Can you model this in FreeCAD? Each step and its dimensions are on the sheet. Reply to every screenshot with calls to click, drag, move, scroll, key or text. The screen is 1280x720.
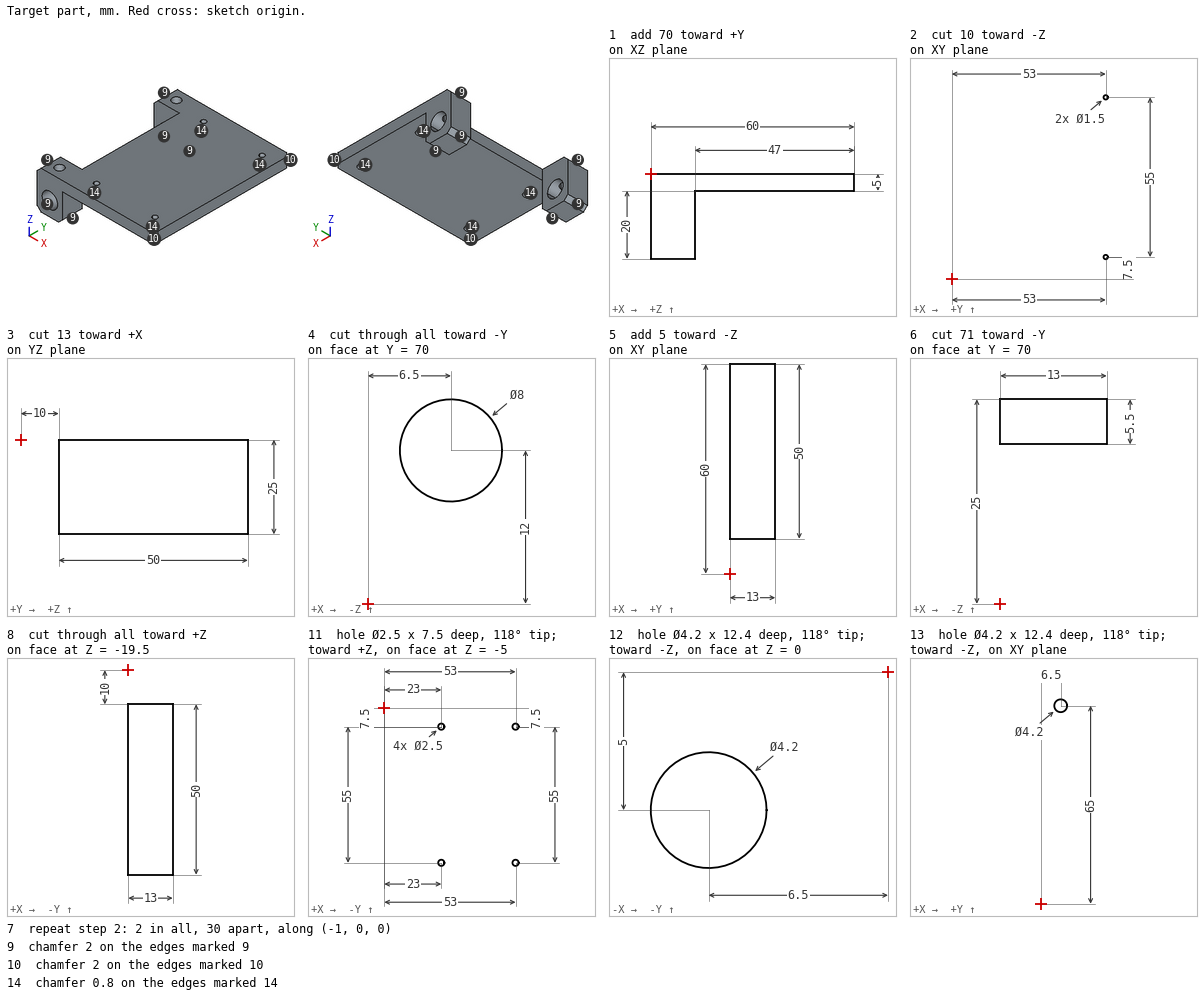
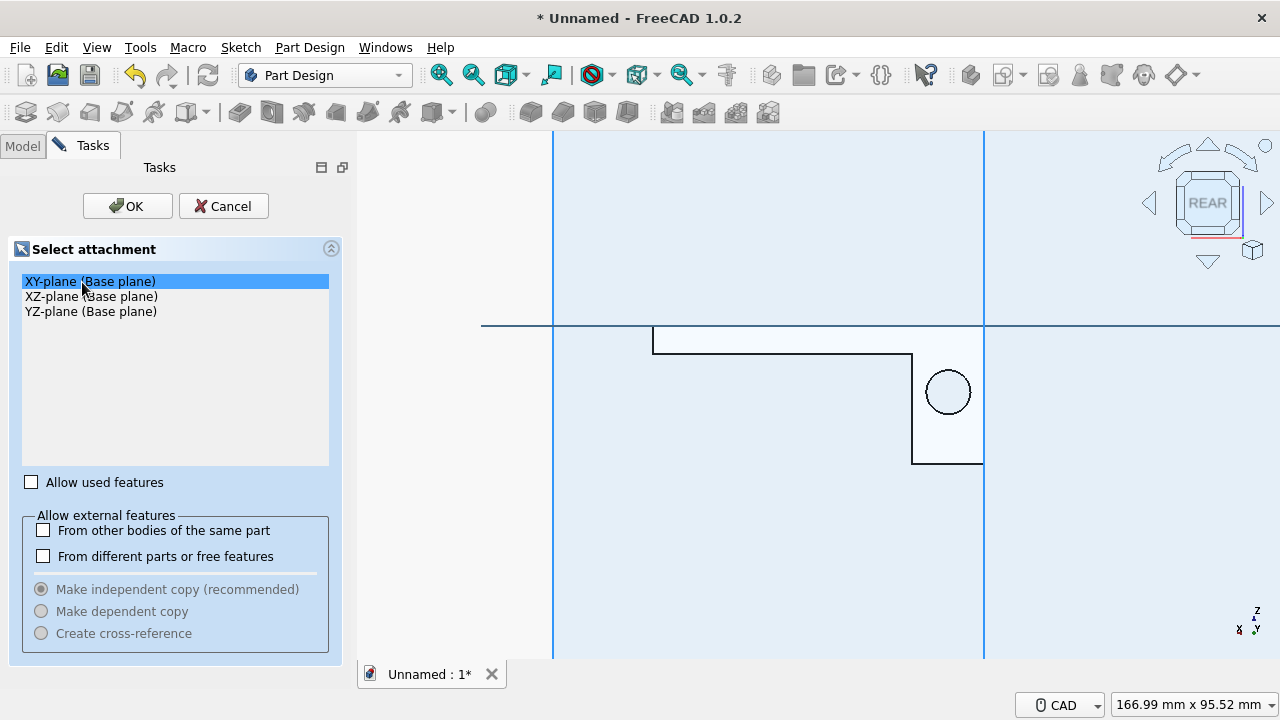
click(128, 206)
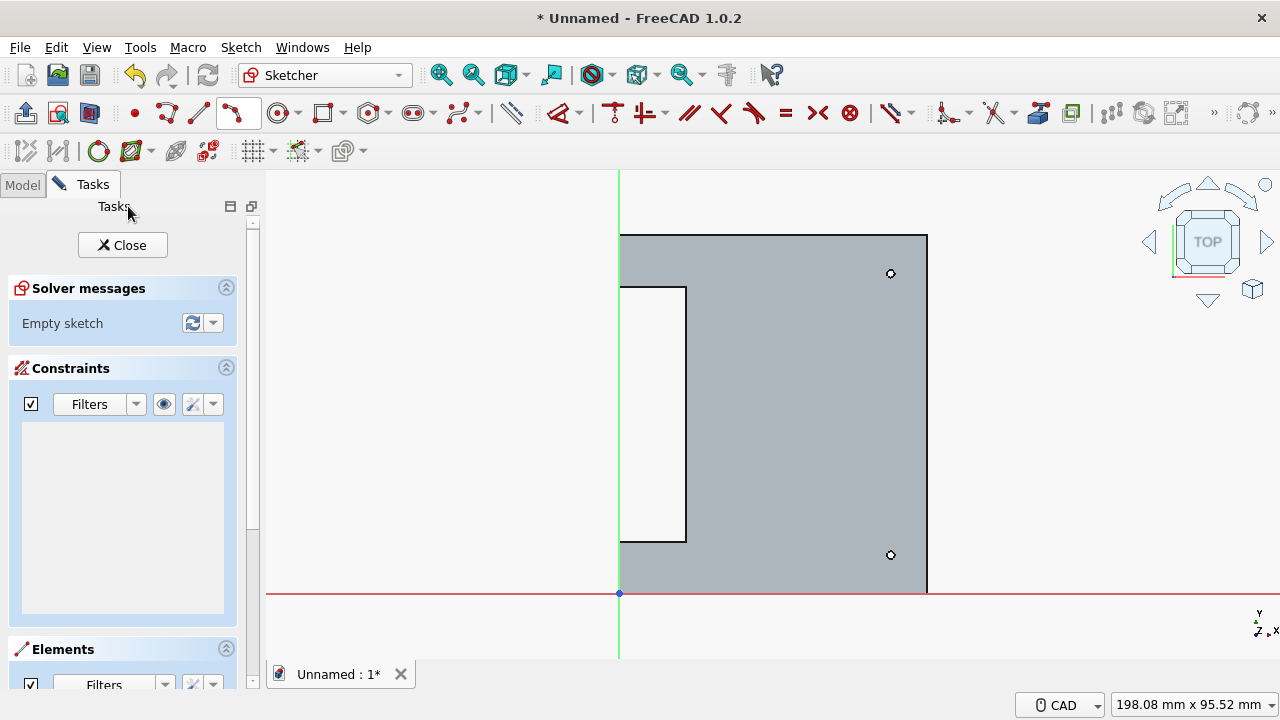
click(324, 114)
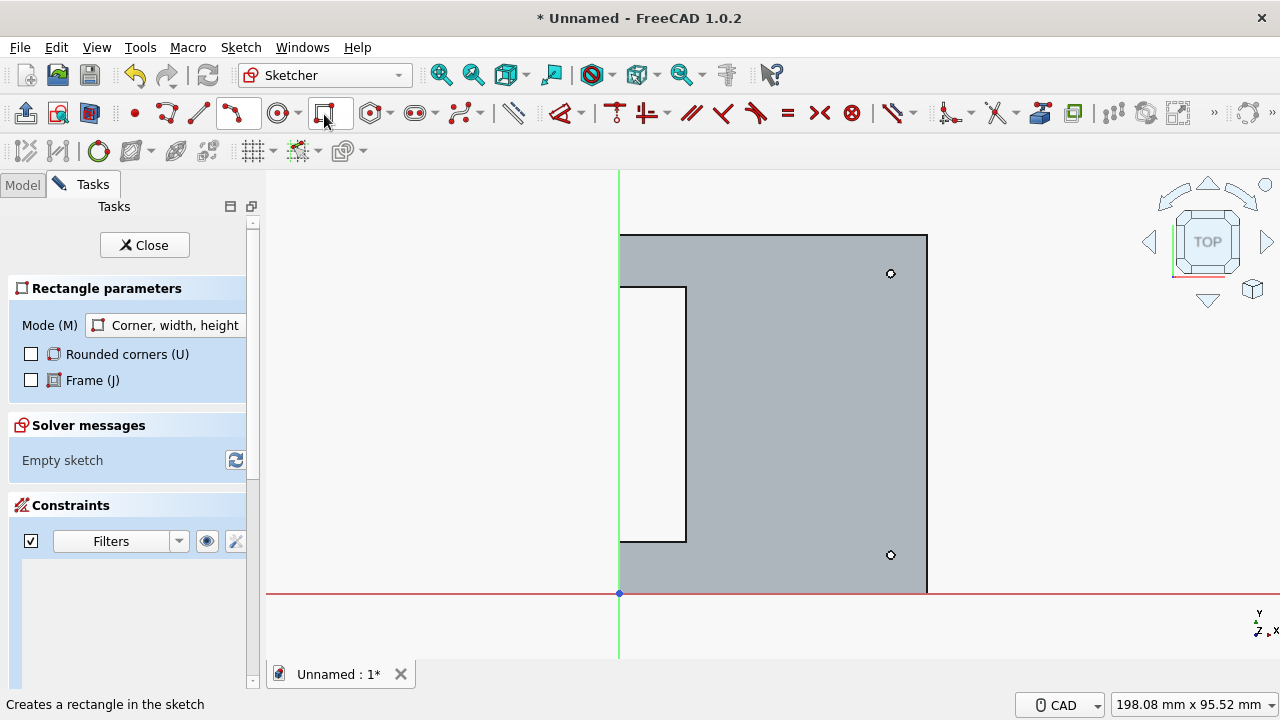
click(619, 287)
move(686, 542)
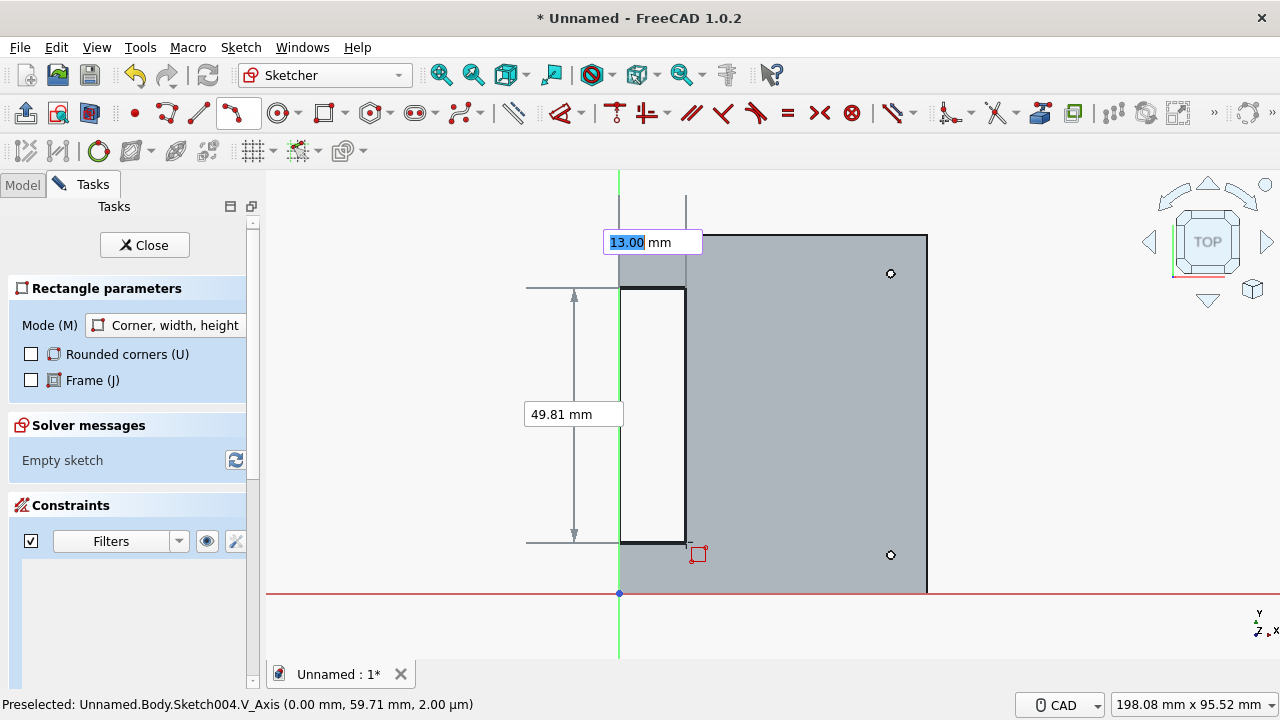
text(13)
key(Tab)
text(50)
key(Return)
key(Escape)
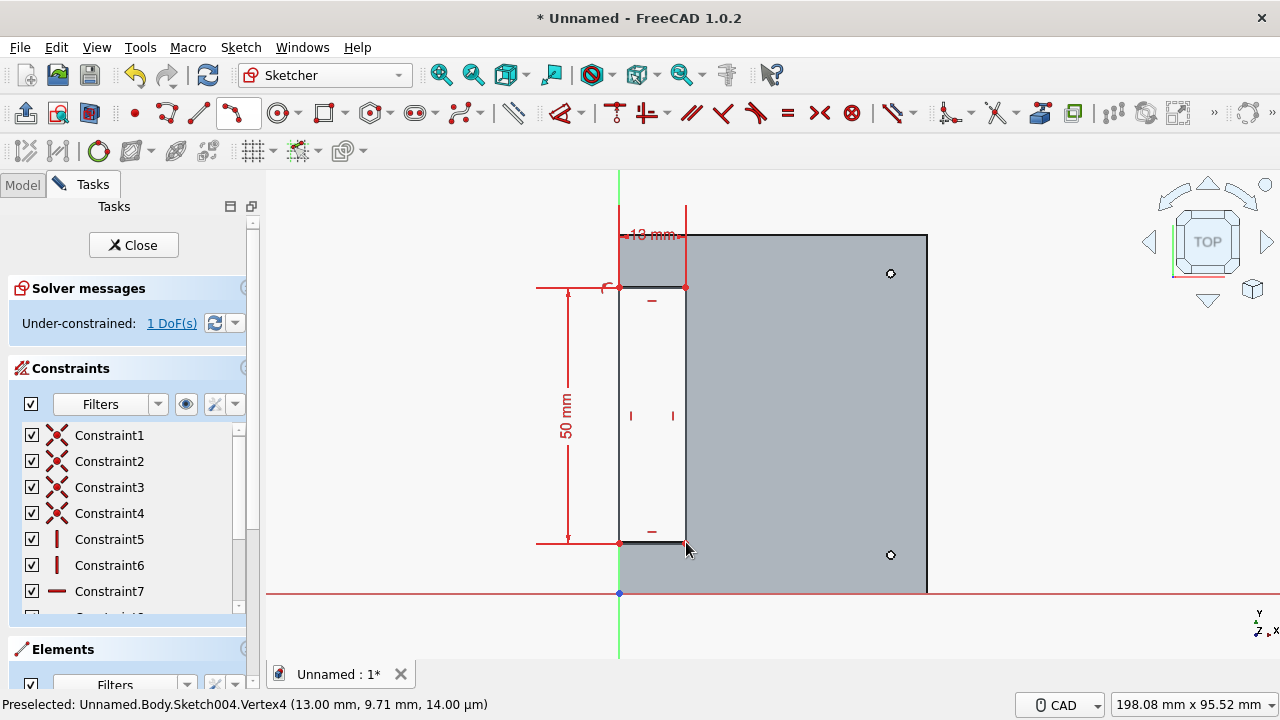
click(560, 114)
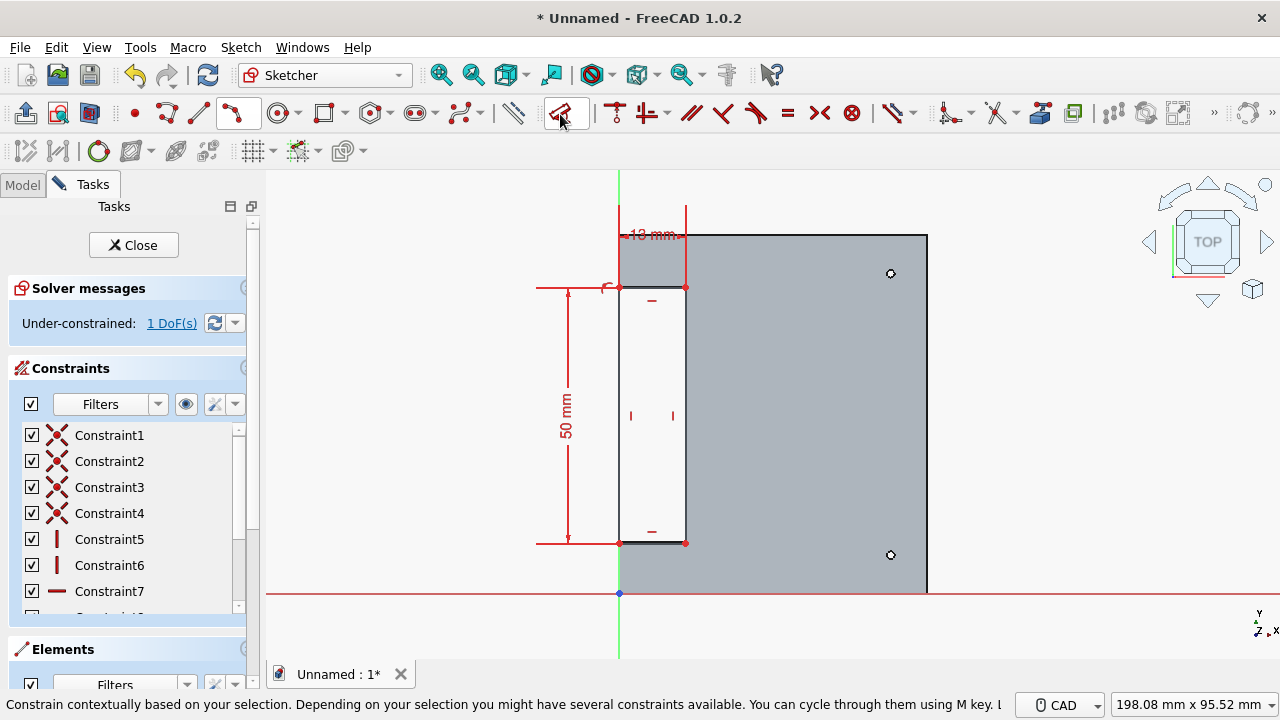
click(619, 288)
click(585, 441)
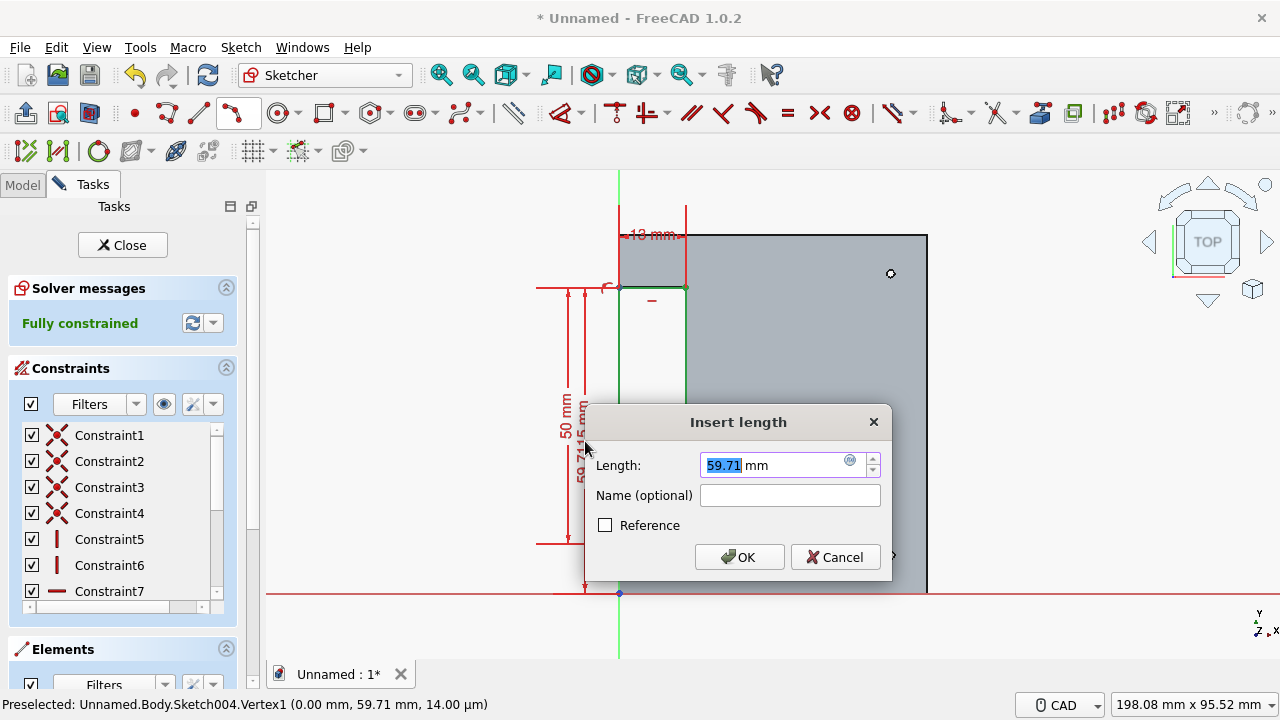
text(60)
key(Return)
key(Escape)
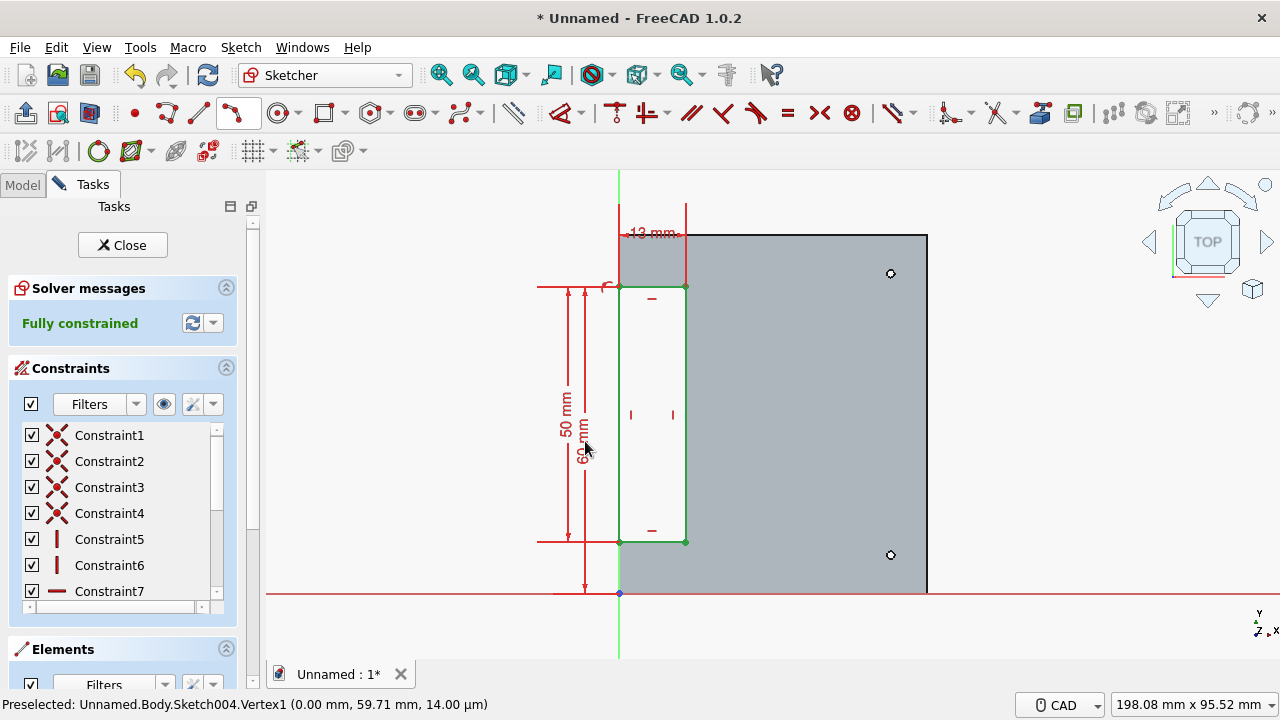
click(123, 245)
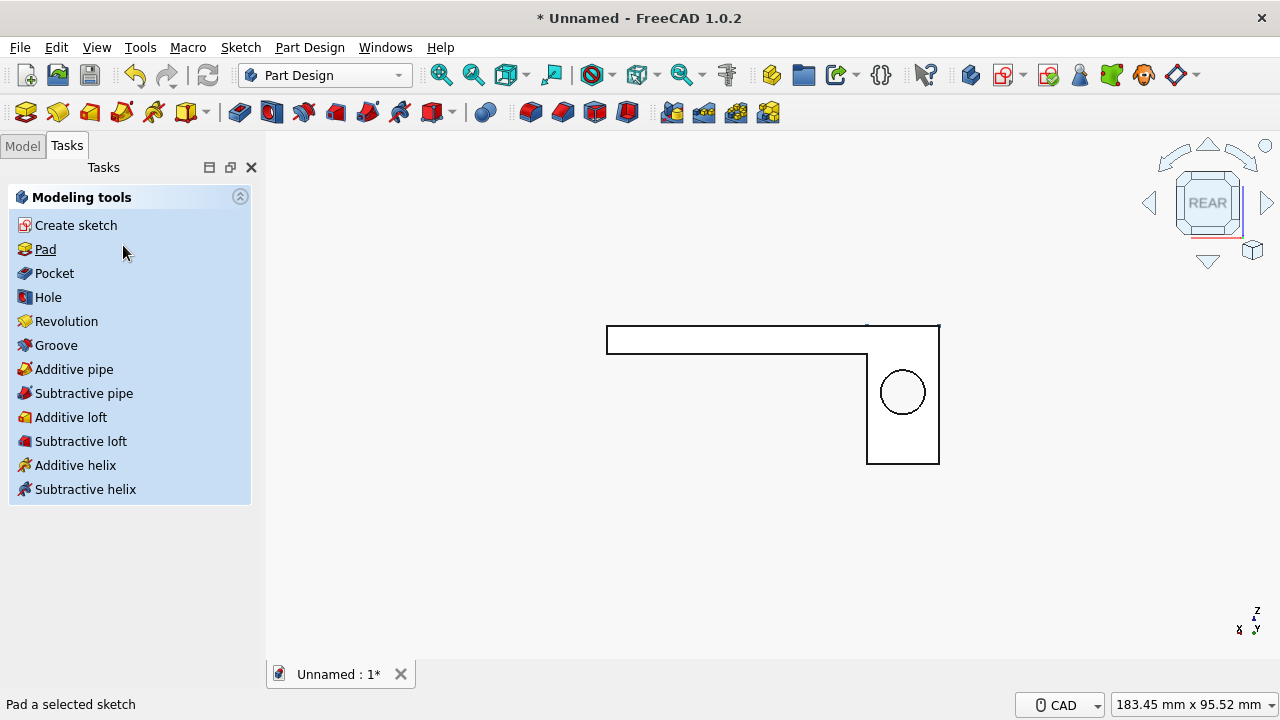
click(26, 112)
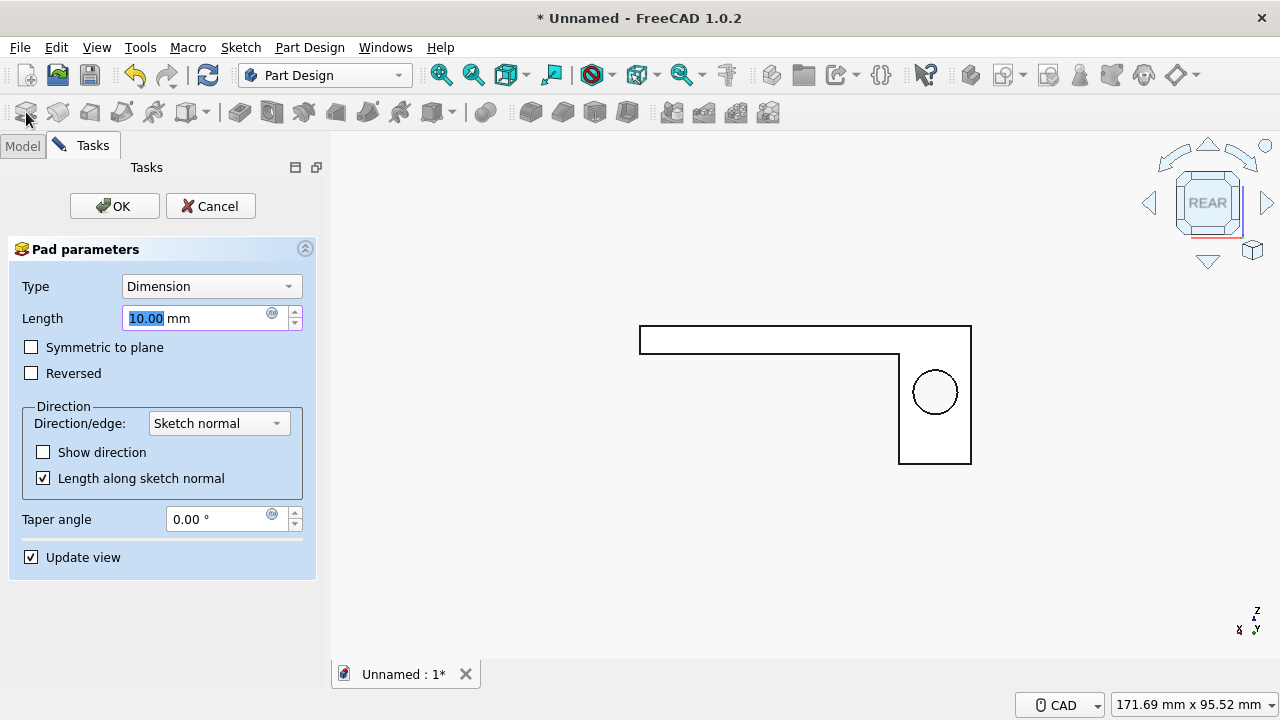
text(5)
key(Tab)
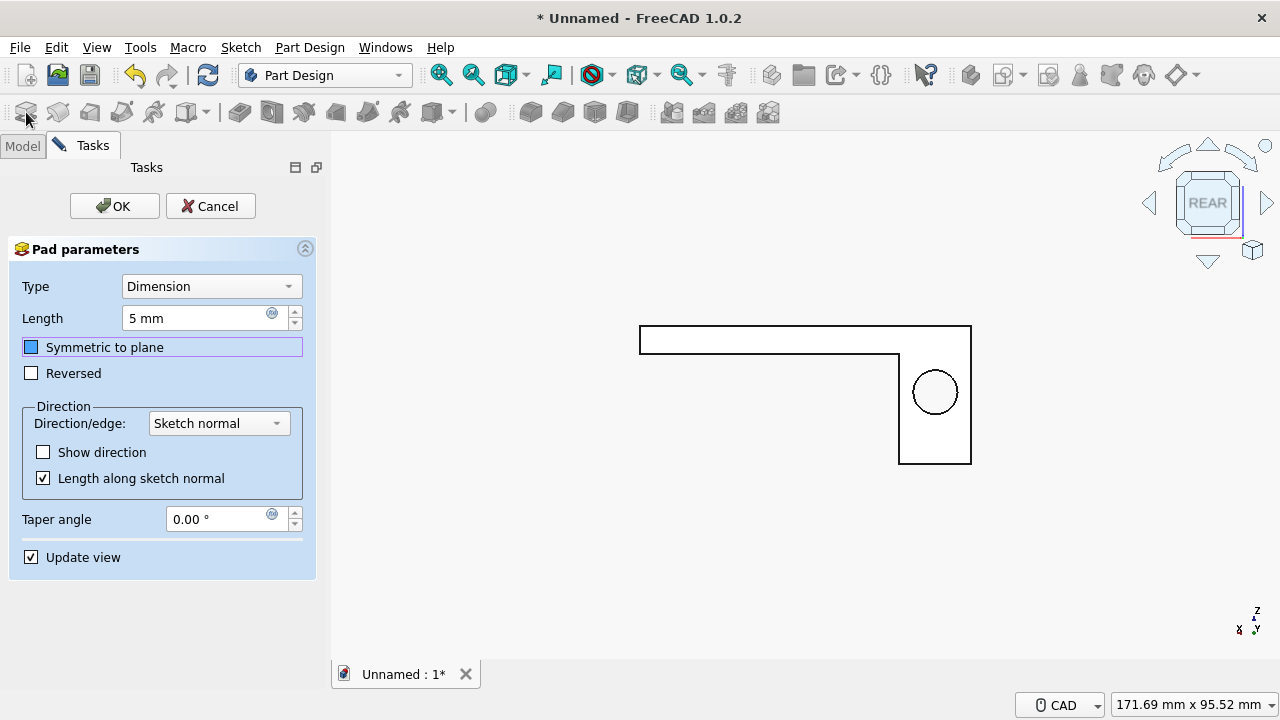
click(30, 373)